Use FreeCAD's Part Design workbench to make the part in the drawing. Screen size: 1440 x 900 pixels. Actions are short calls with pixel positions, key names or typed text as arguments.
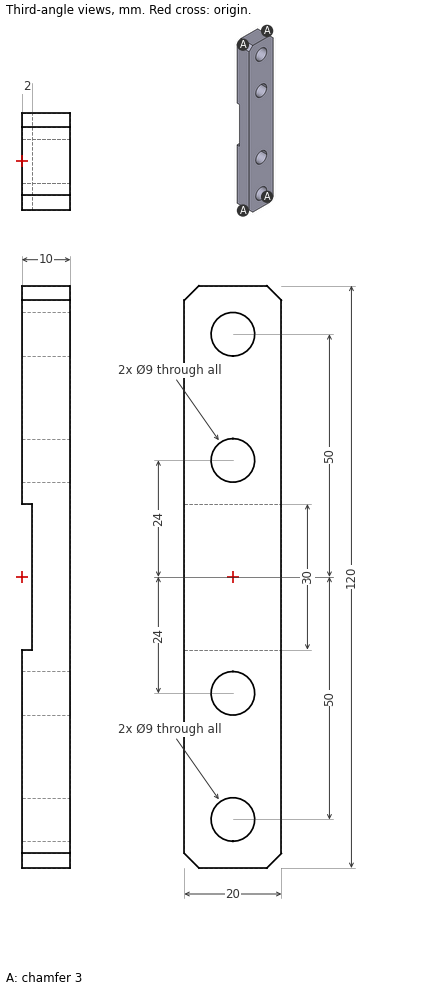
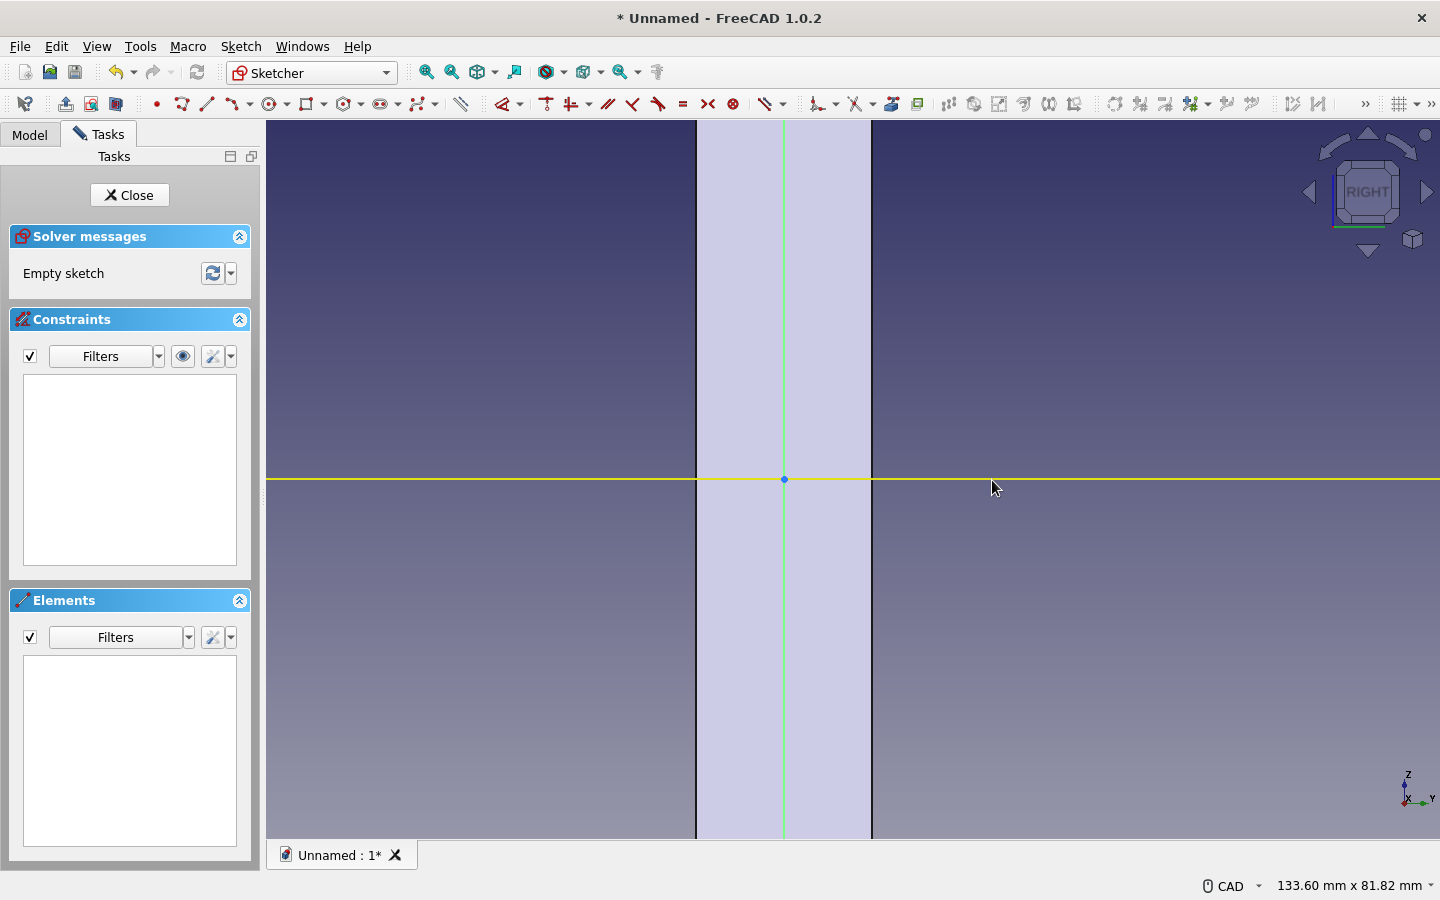
key(g)
key(c)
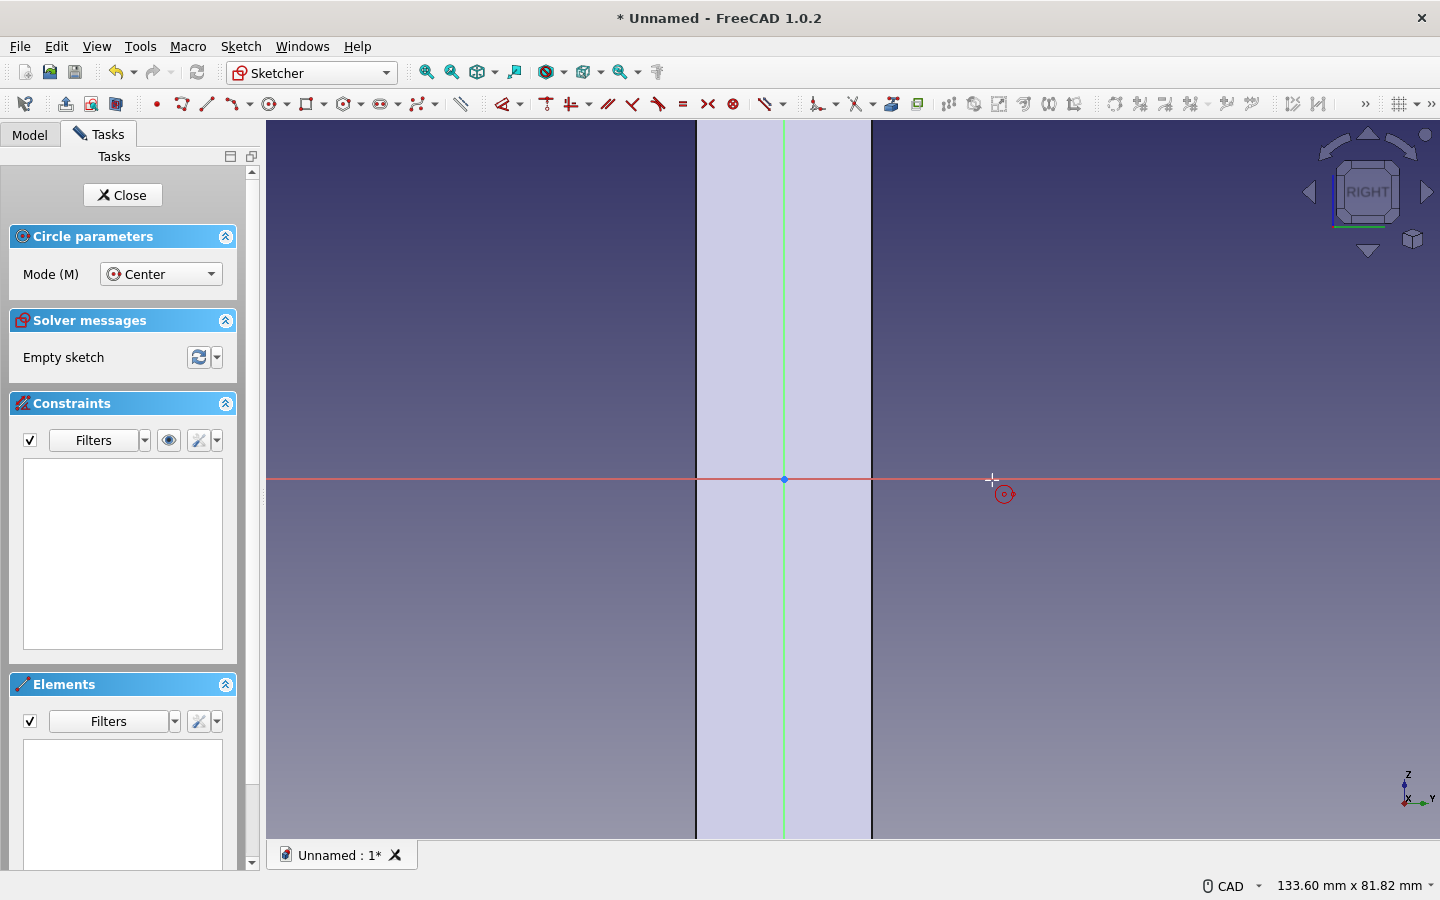
click(784, 268)
move(812, 240)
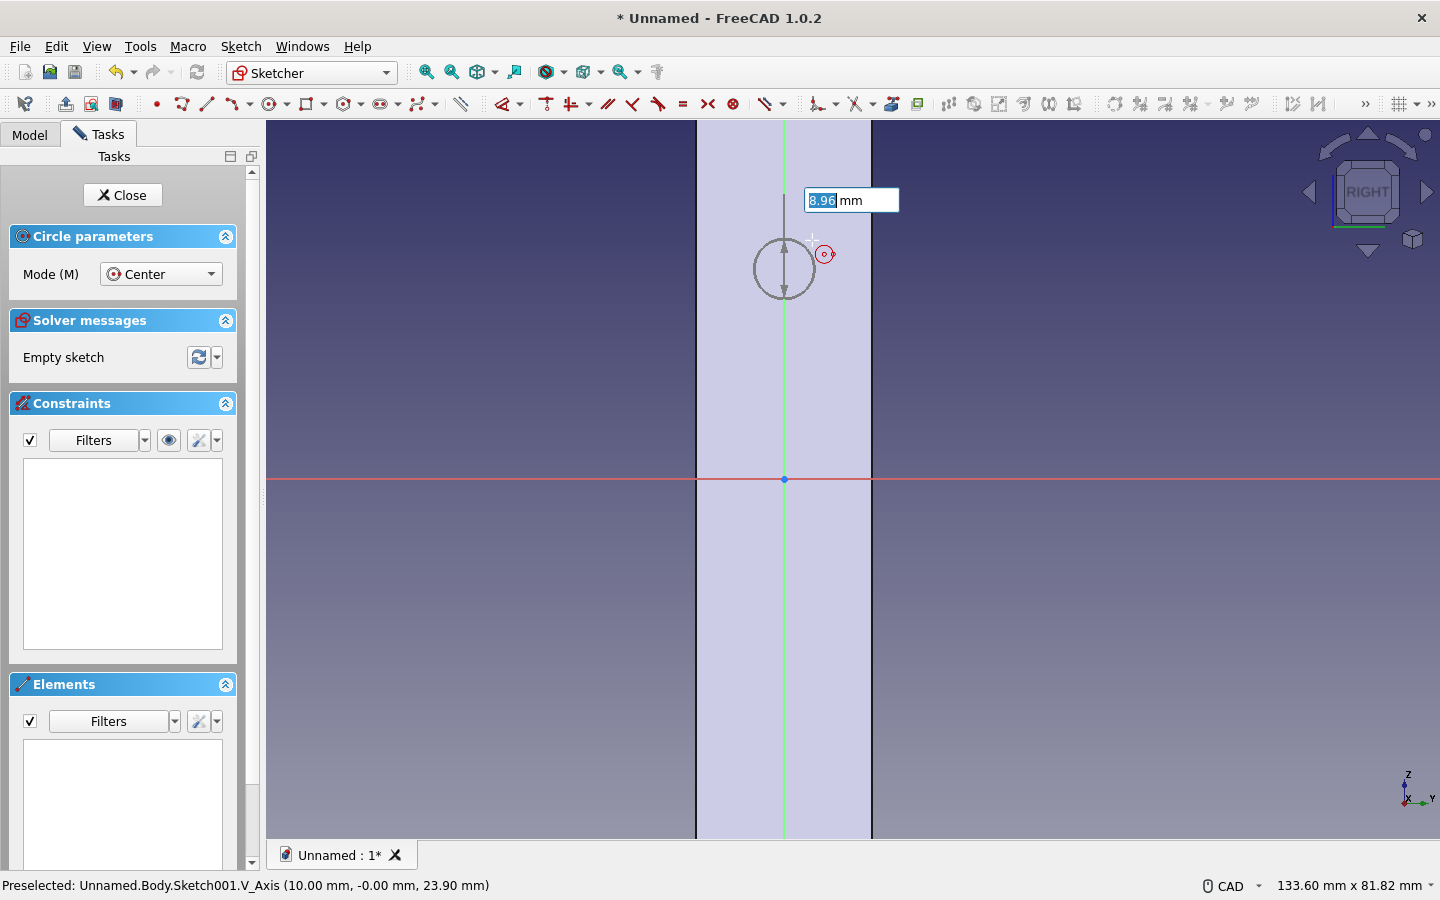
text(9)
key(Return)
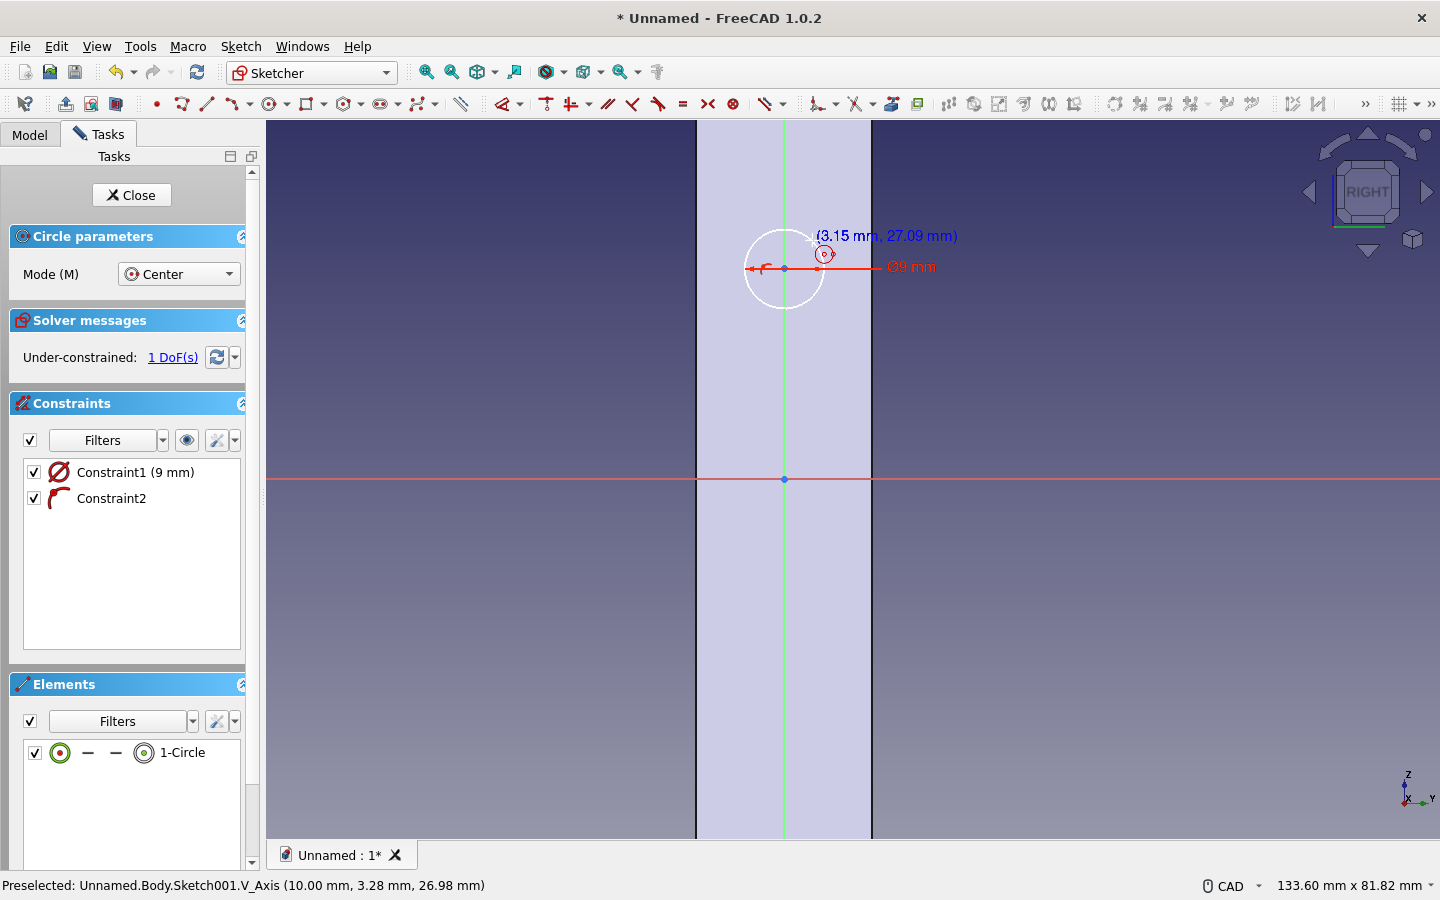
click(784, 690)
move(812, 662)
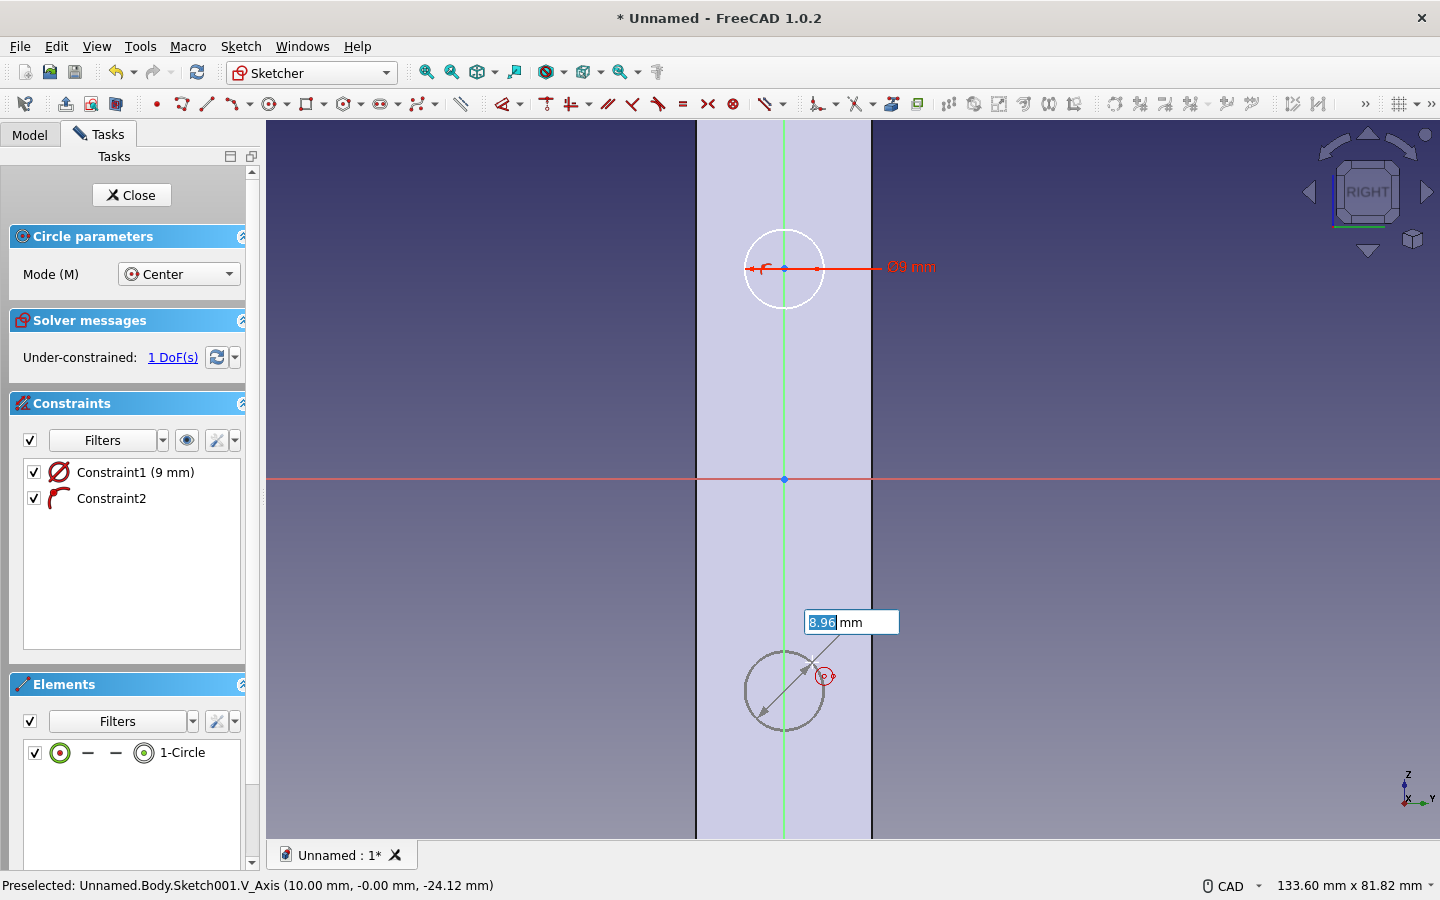
text(9)
key(Return)
key(Escape)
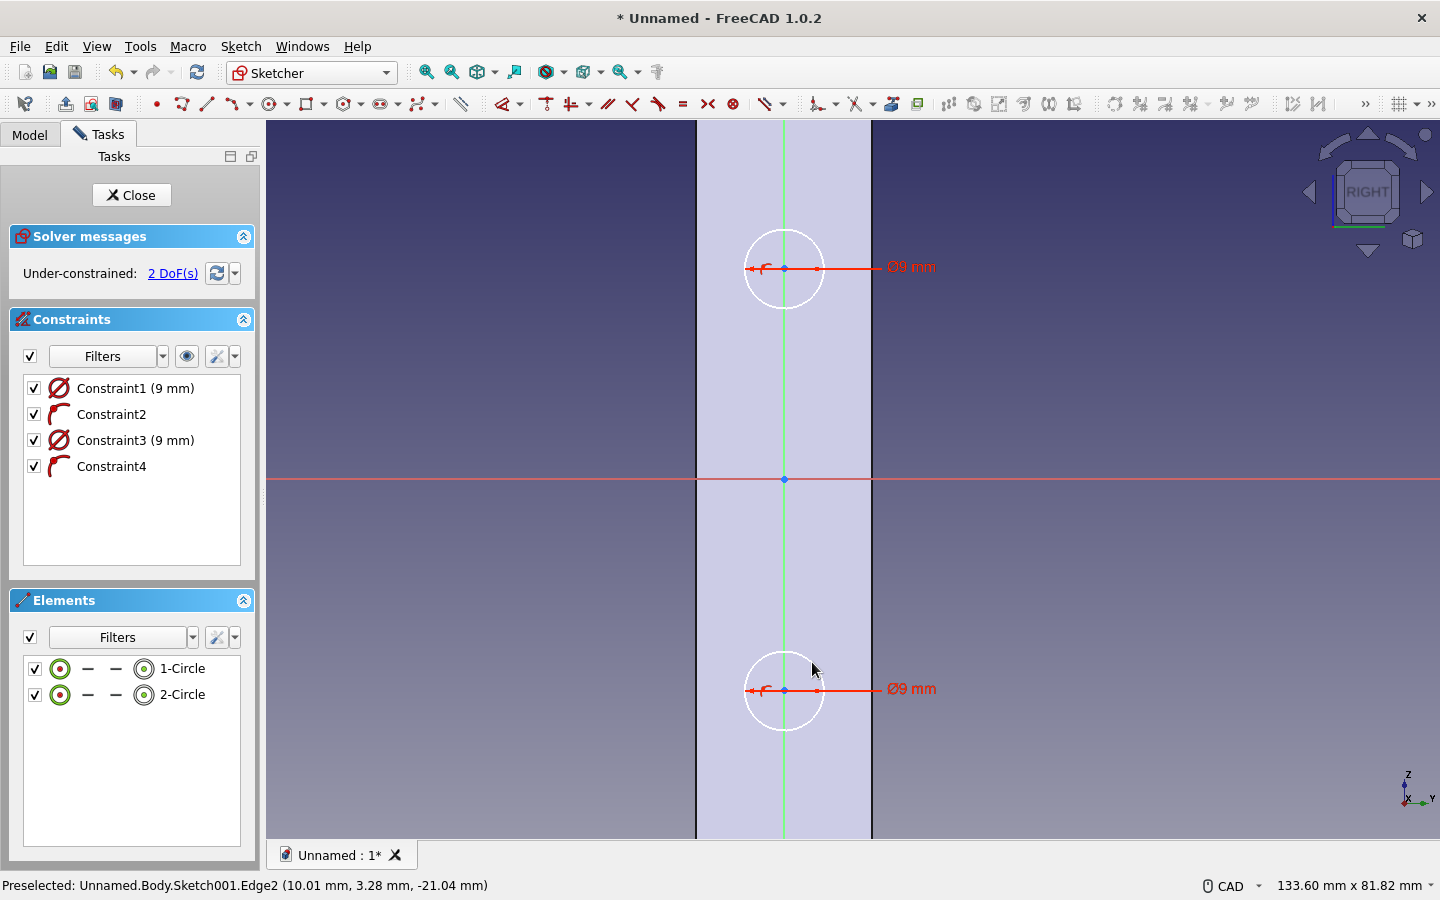
click(502, 104)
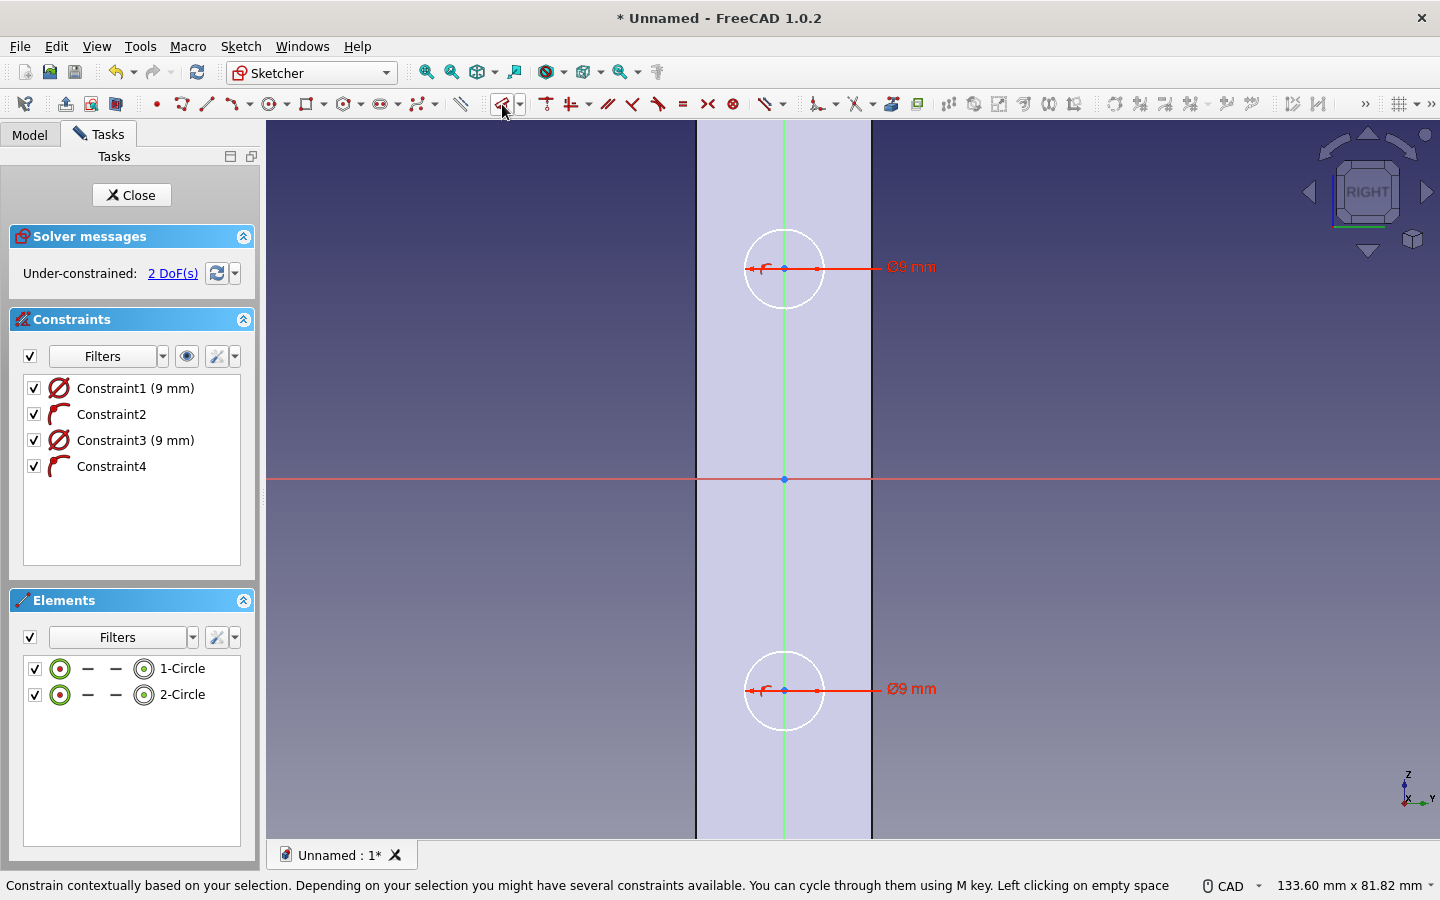
click(784, 269)
click(818, 374)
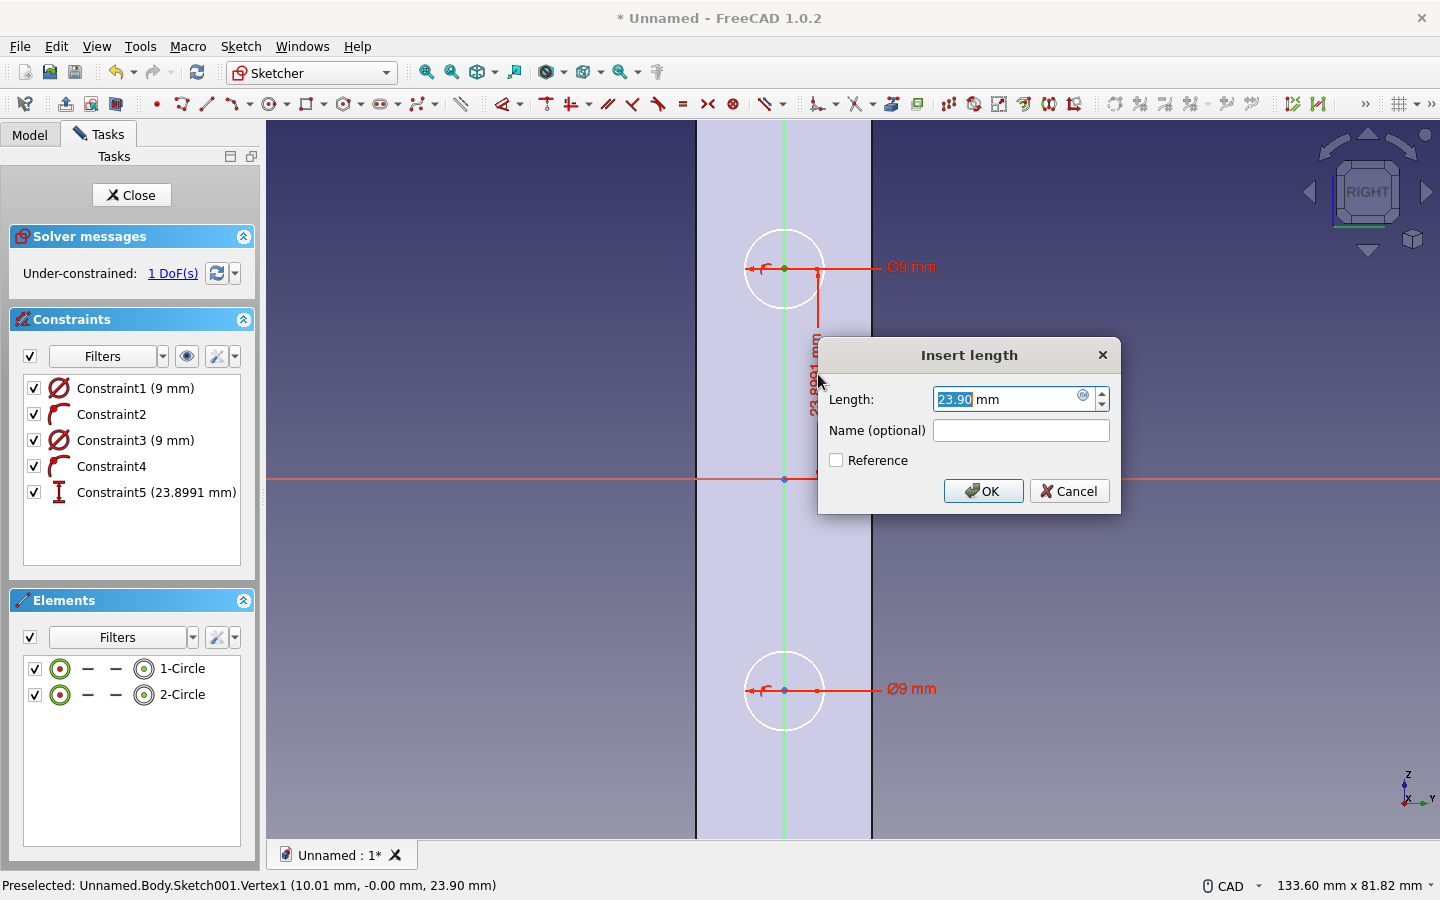
text(24)
key(Return)